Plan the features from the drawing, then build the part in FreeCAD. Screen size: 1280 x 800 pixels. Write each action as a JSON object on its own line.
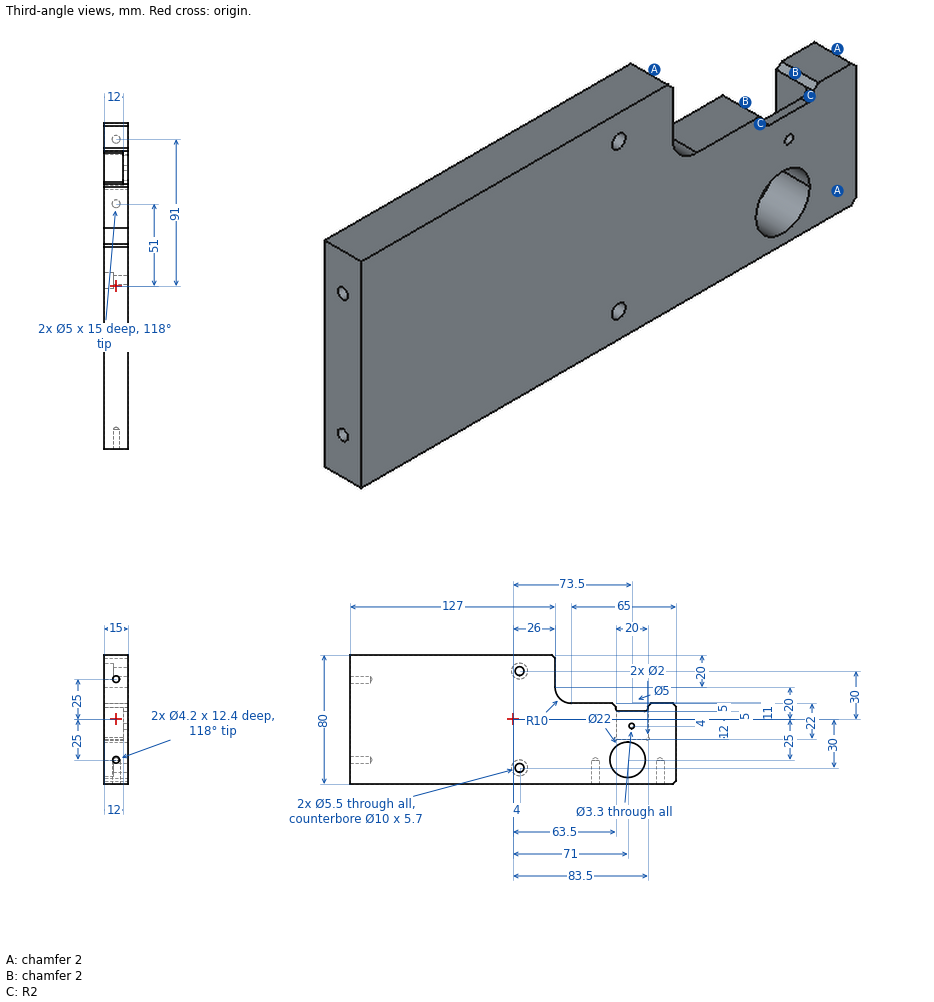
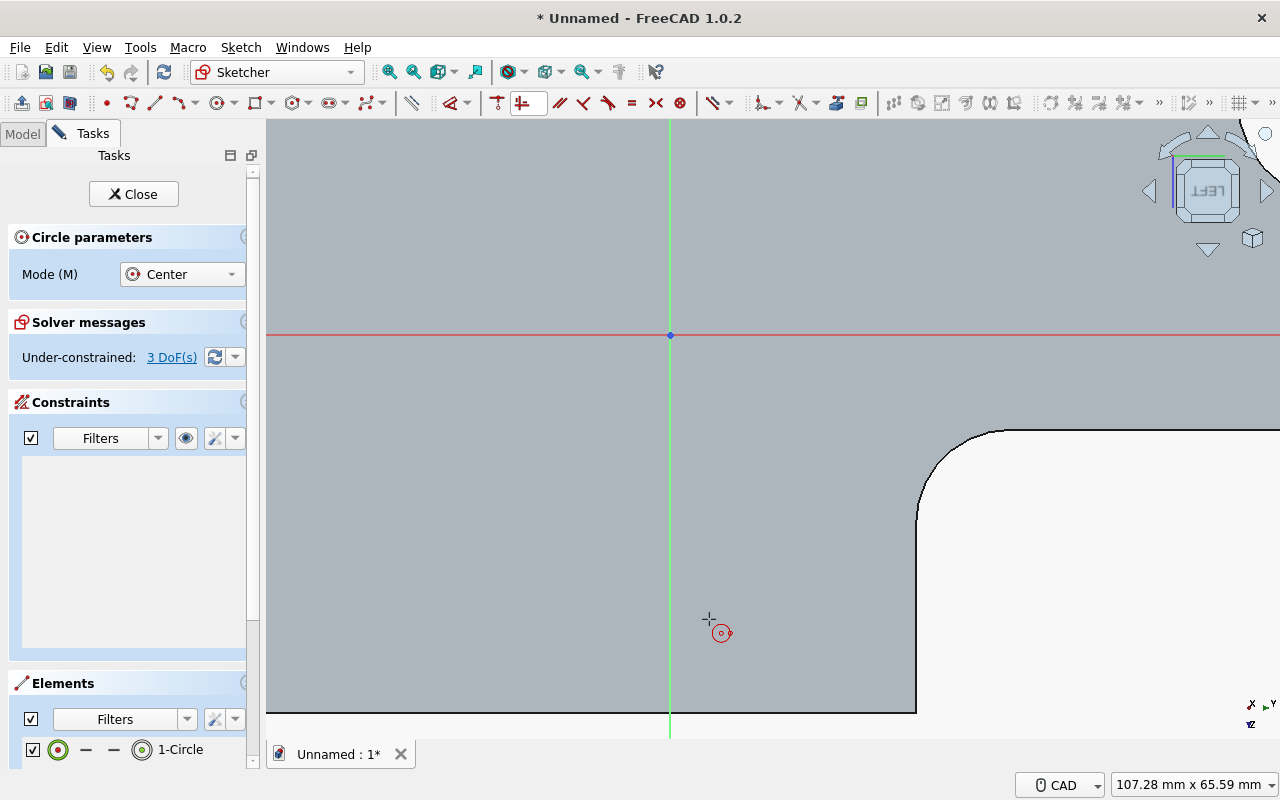
{"action": "left_click", "coordinate": [708, 619]}
{"action": "left_click", "coordinate": [726, 600]}
{"action": "key", "text": "Escape"}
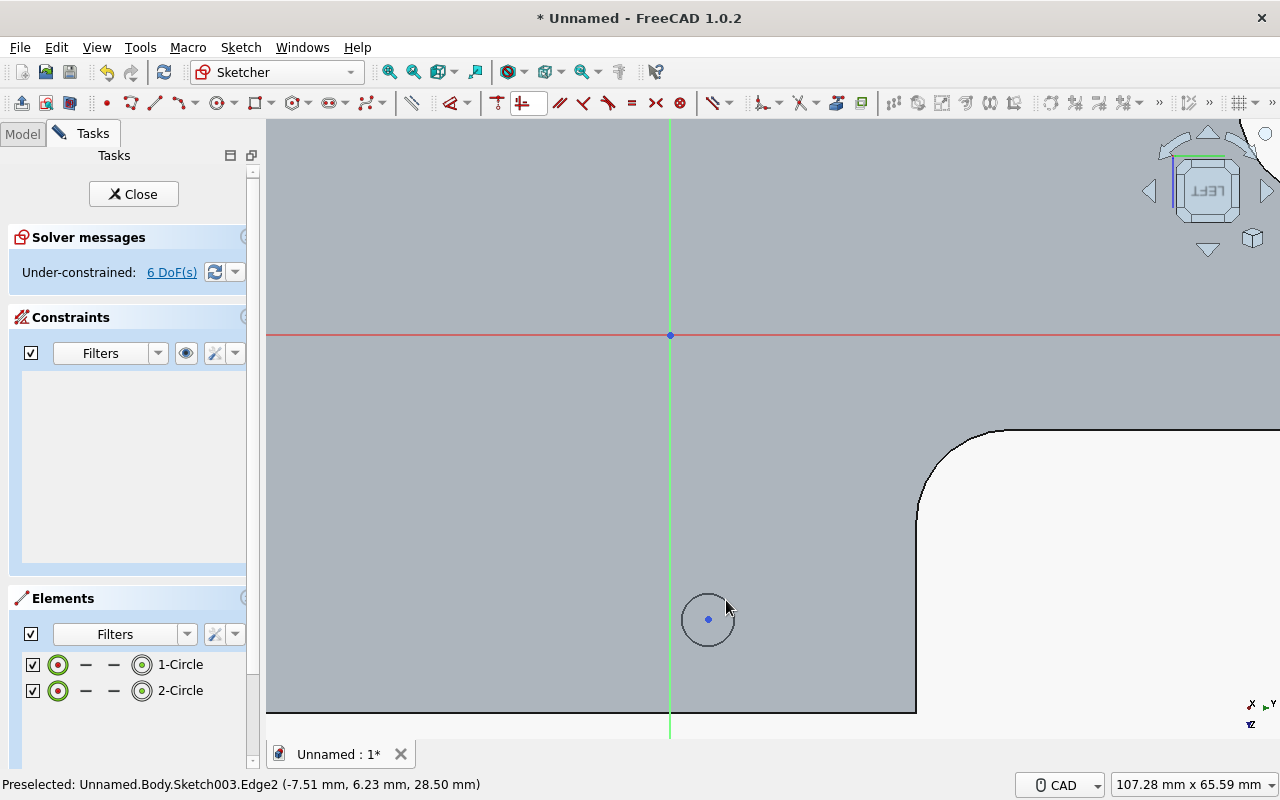
{"action": "scroll", "coordinate": [709, 620], "scroll_direction": "down", "scroll_amount": 2}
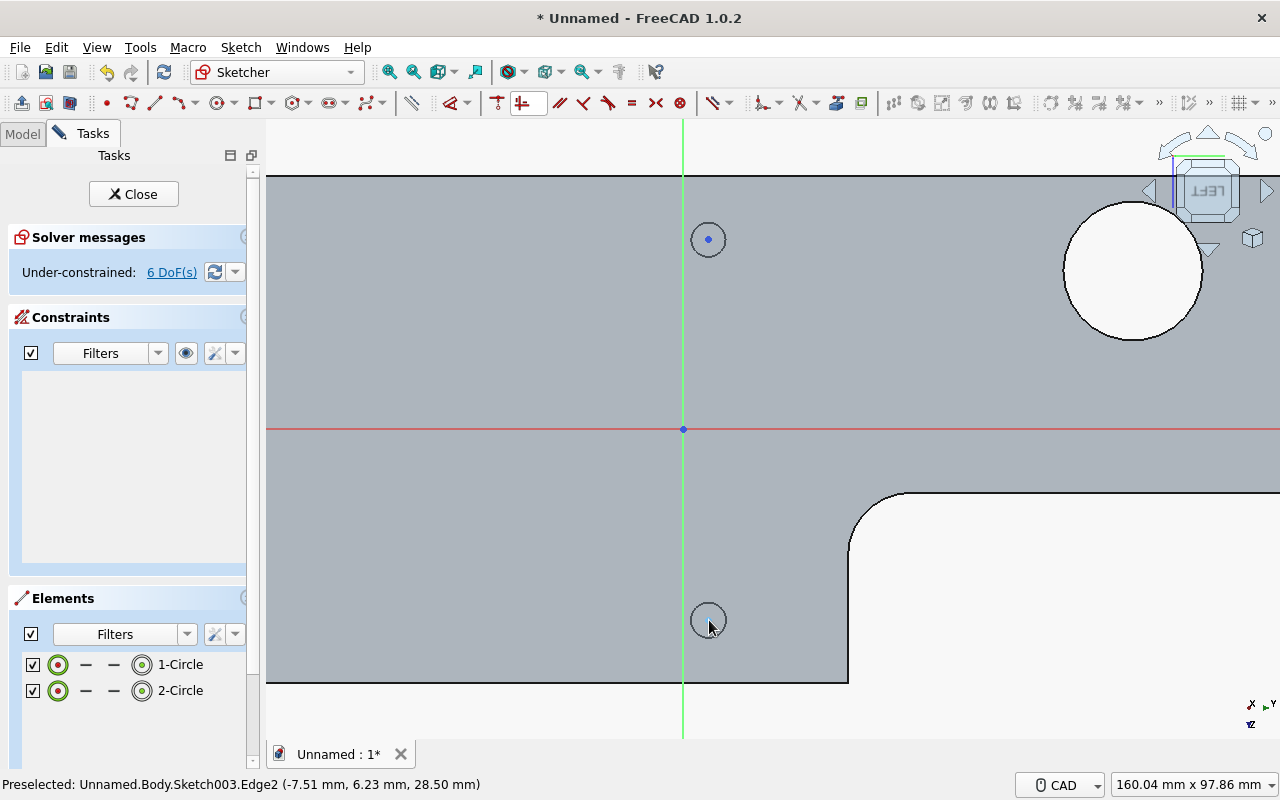
{"action": "left_click", "coordinate": [721, 228]}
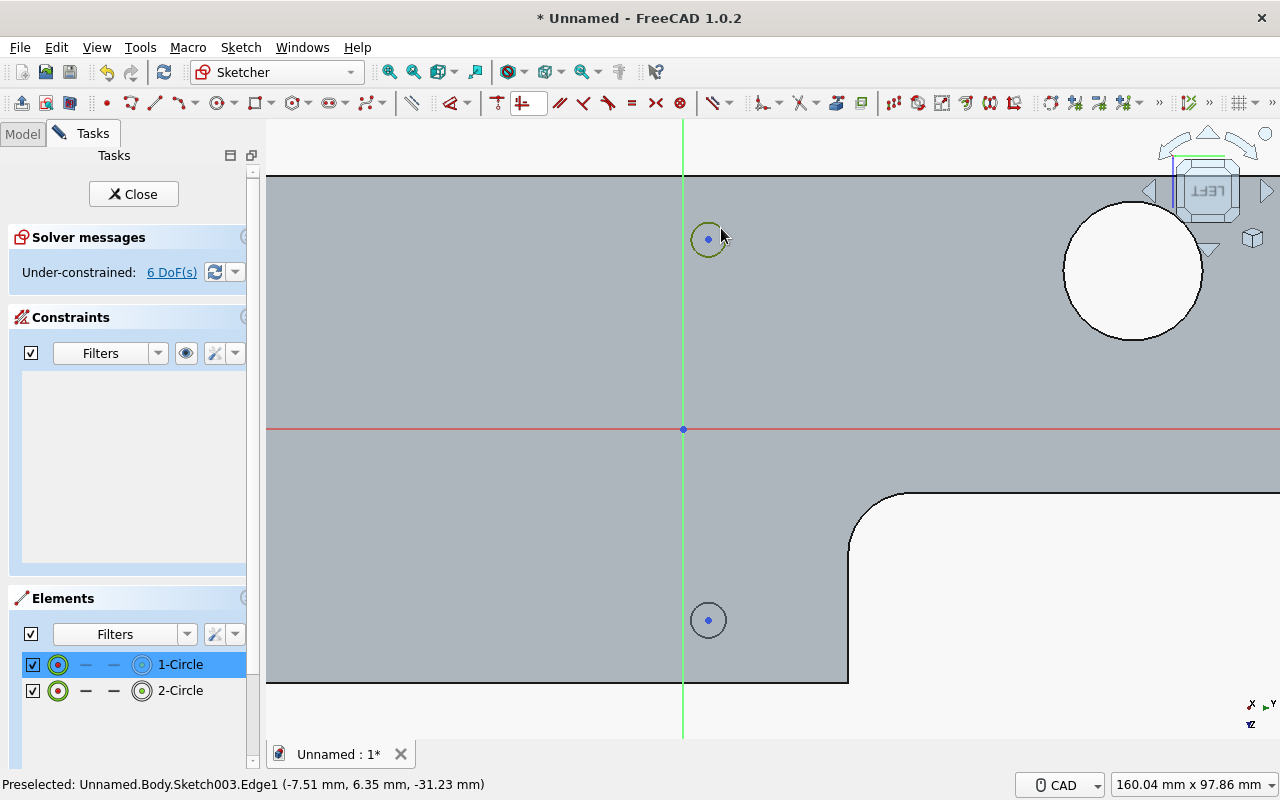
{"action": "left_click", "coordinate": [721, 608]}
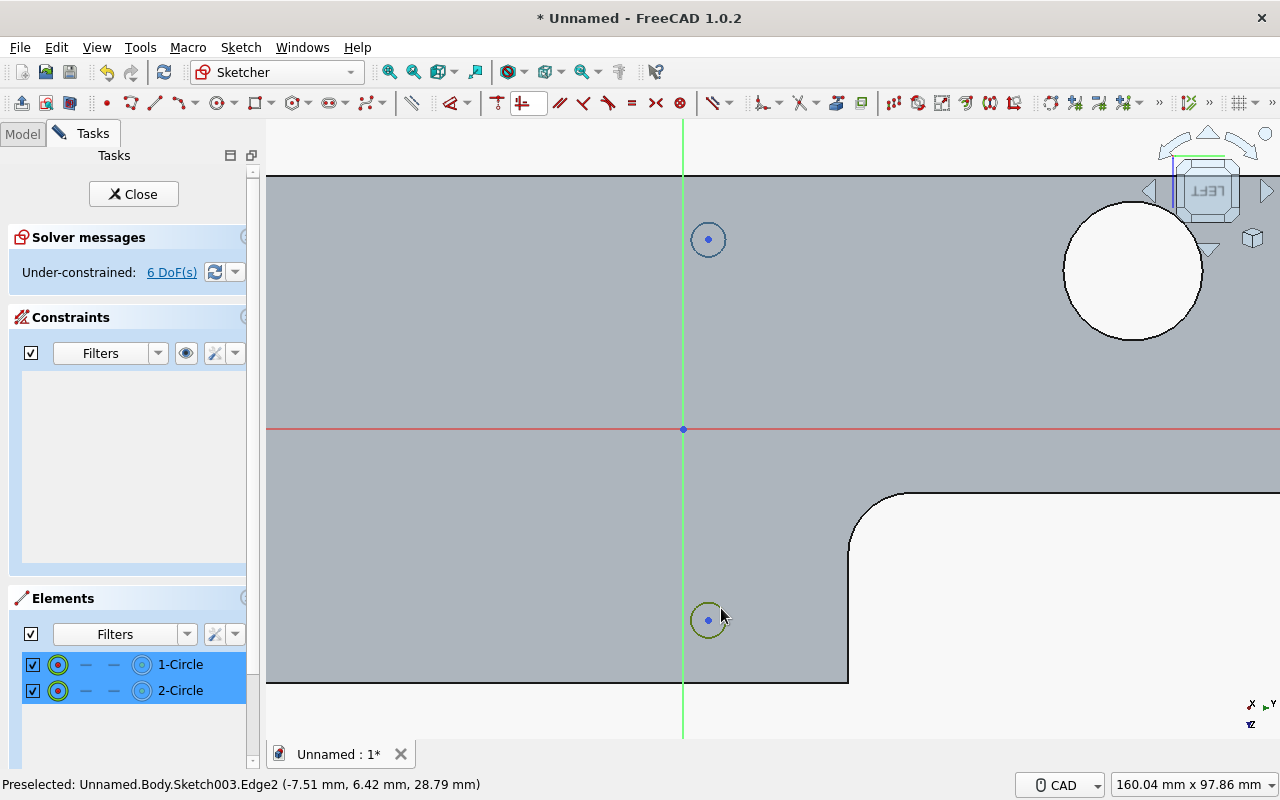
{"action": "left_click", "coordinate": [632, 104]}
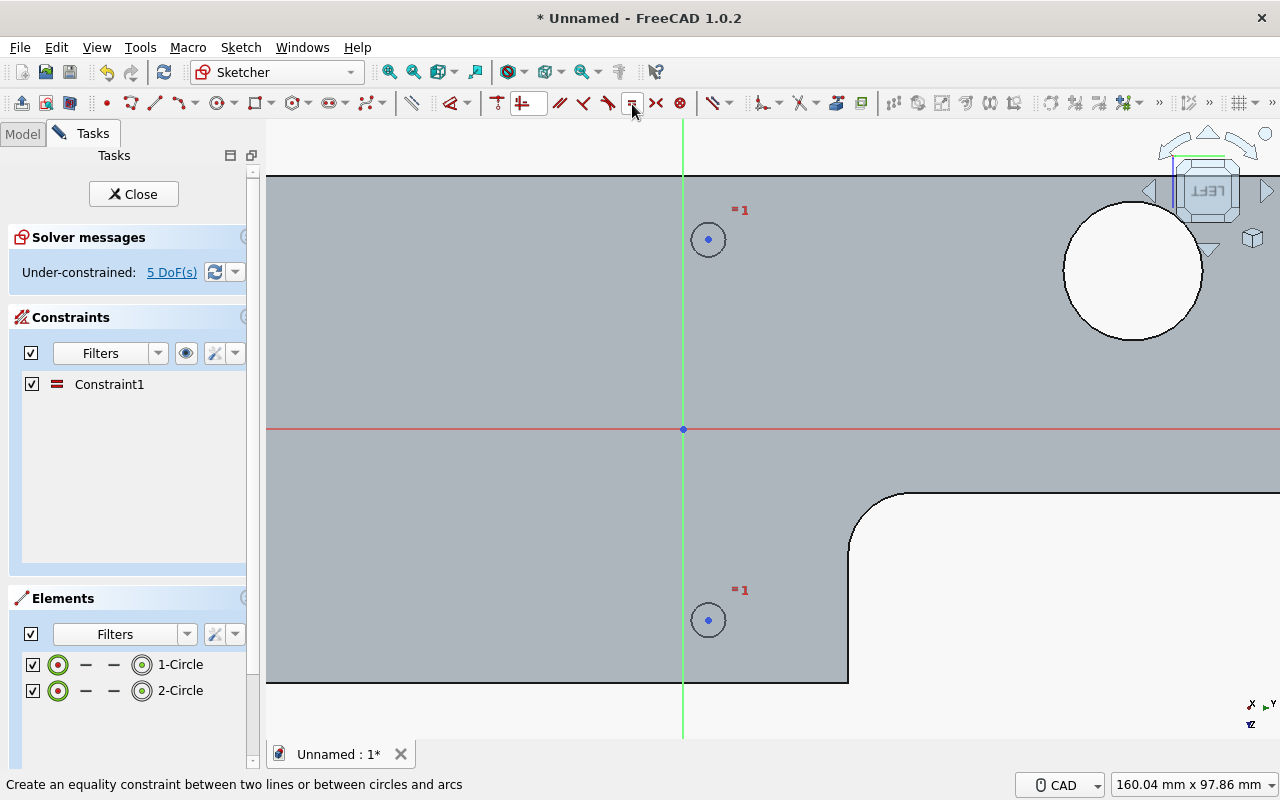
{"action": "left_click", "coordinate": [708, 240]}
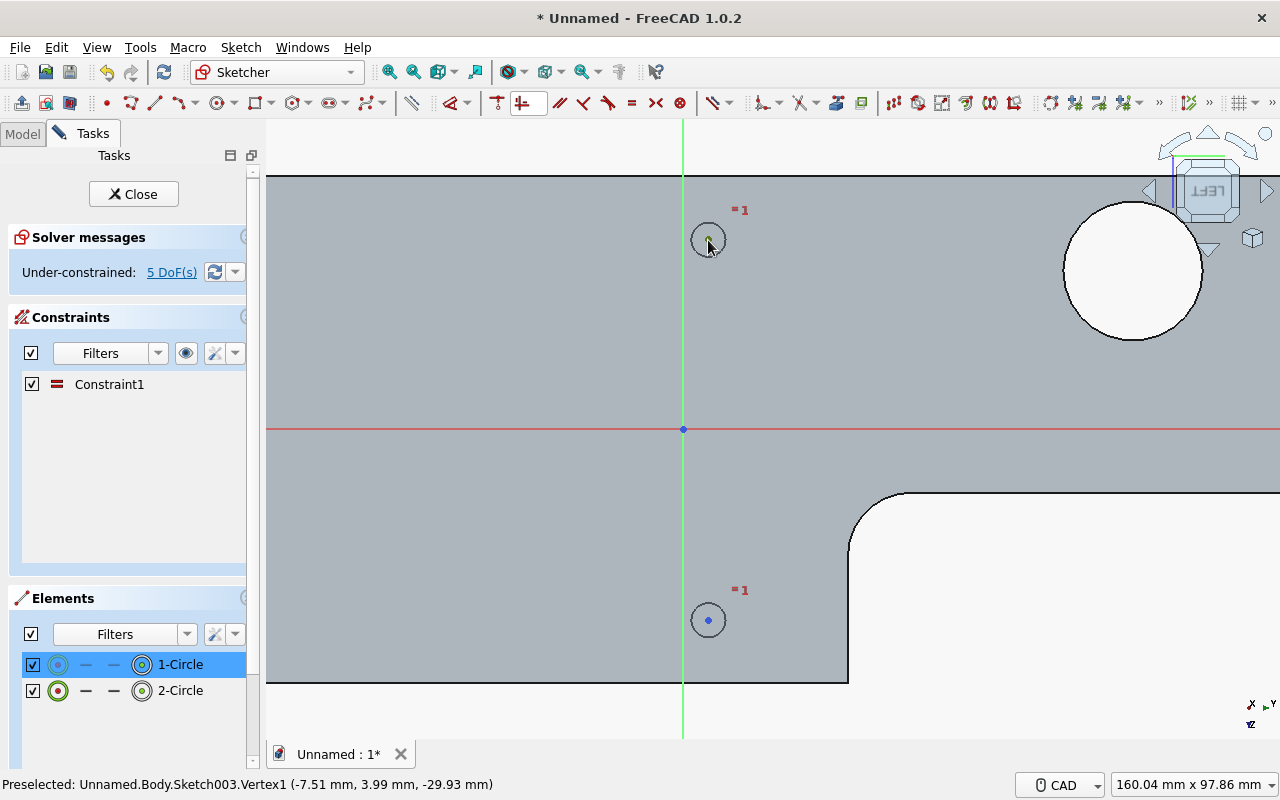
{"action": "left_click", "coordinate": [708, 620]}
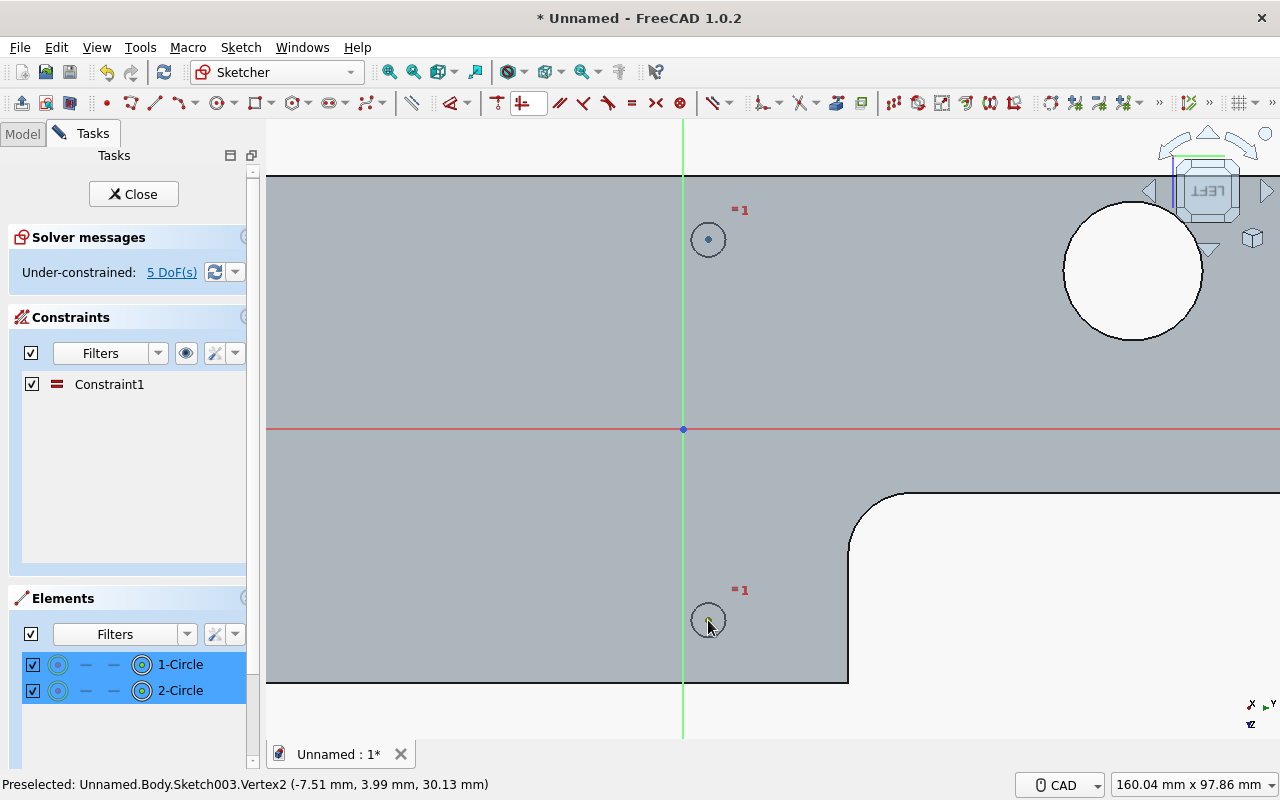
{"action": "key", "text": "v"}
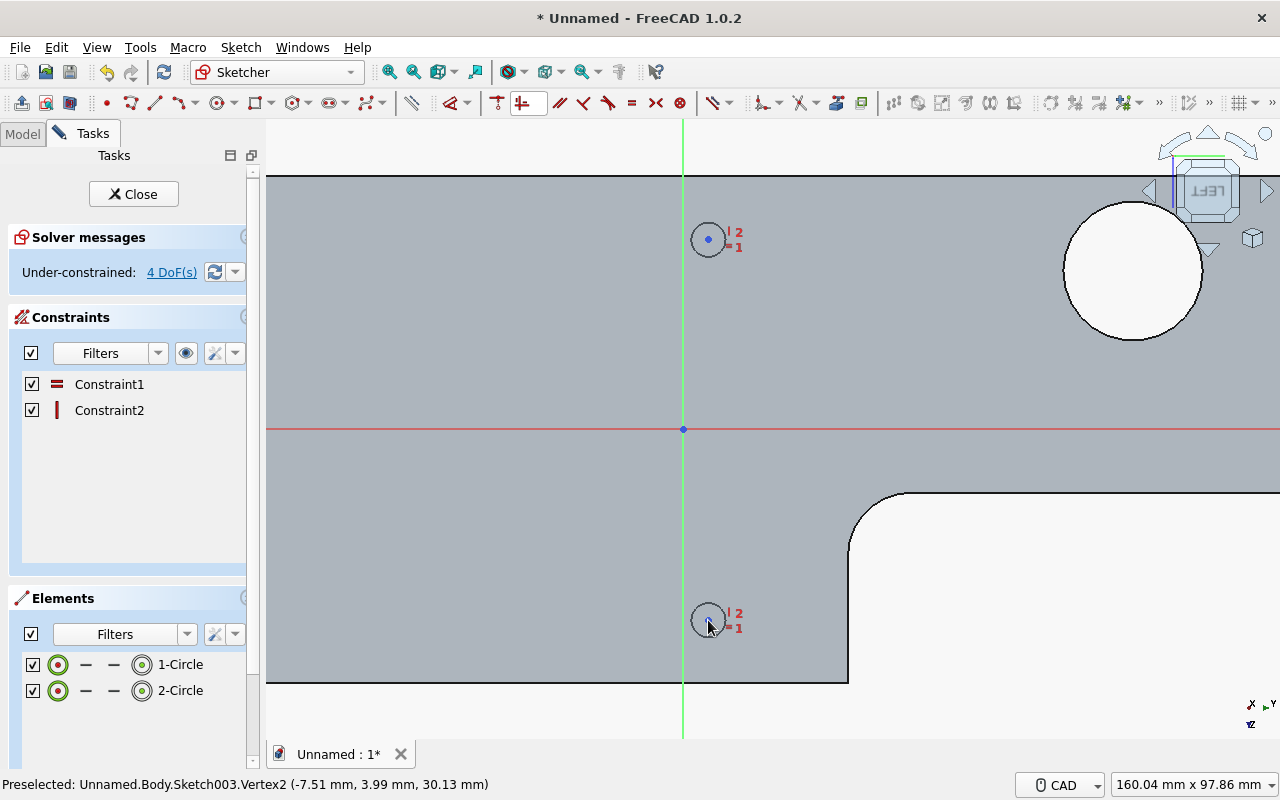
{"action": "left_click", "coordinate": [450, 104]}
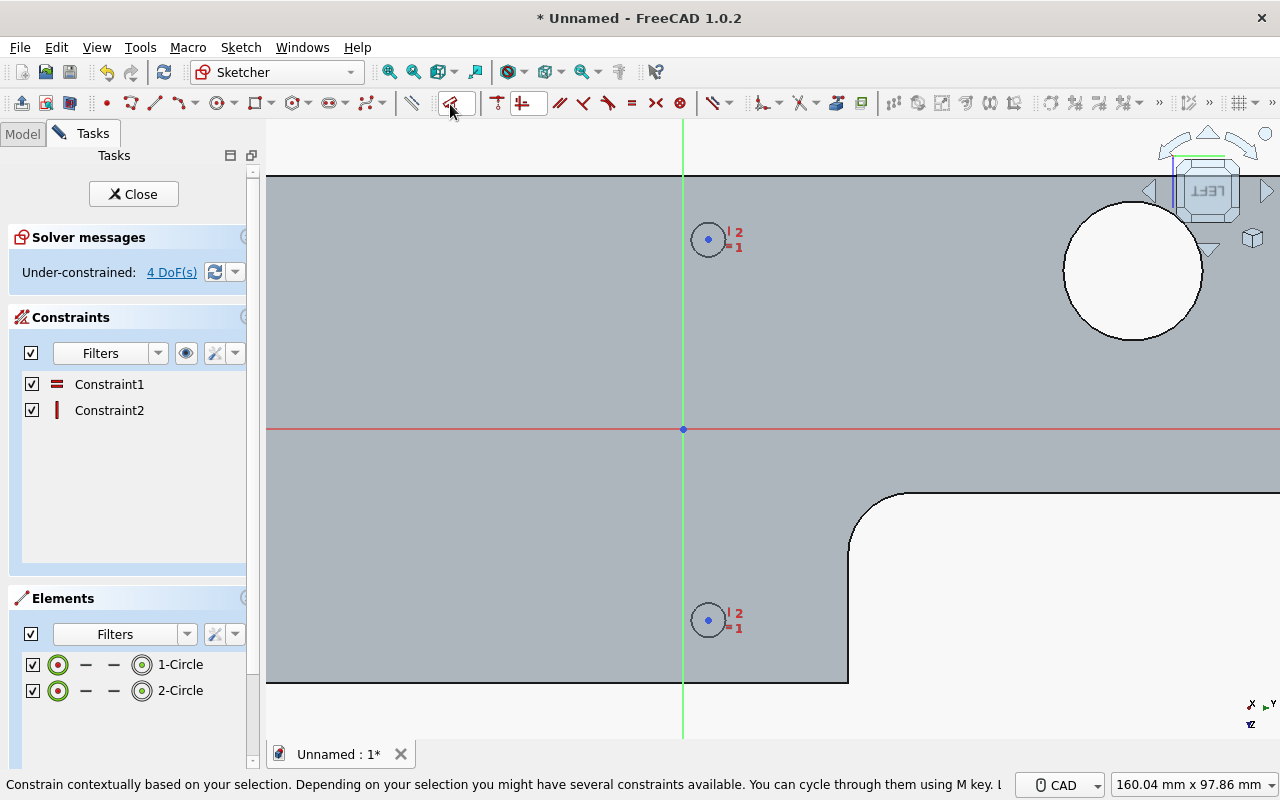
{"action": "left_click", "coordinate": [721, 228]}
{"action": "left_click", "coordinate": [744, 206]}